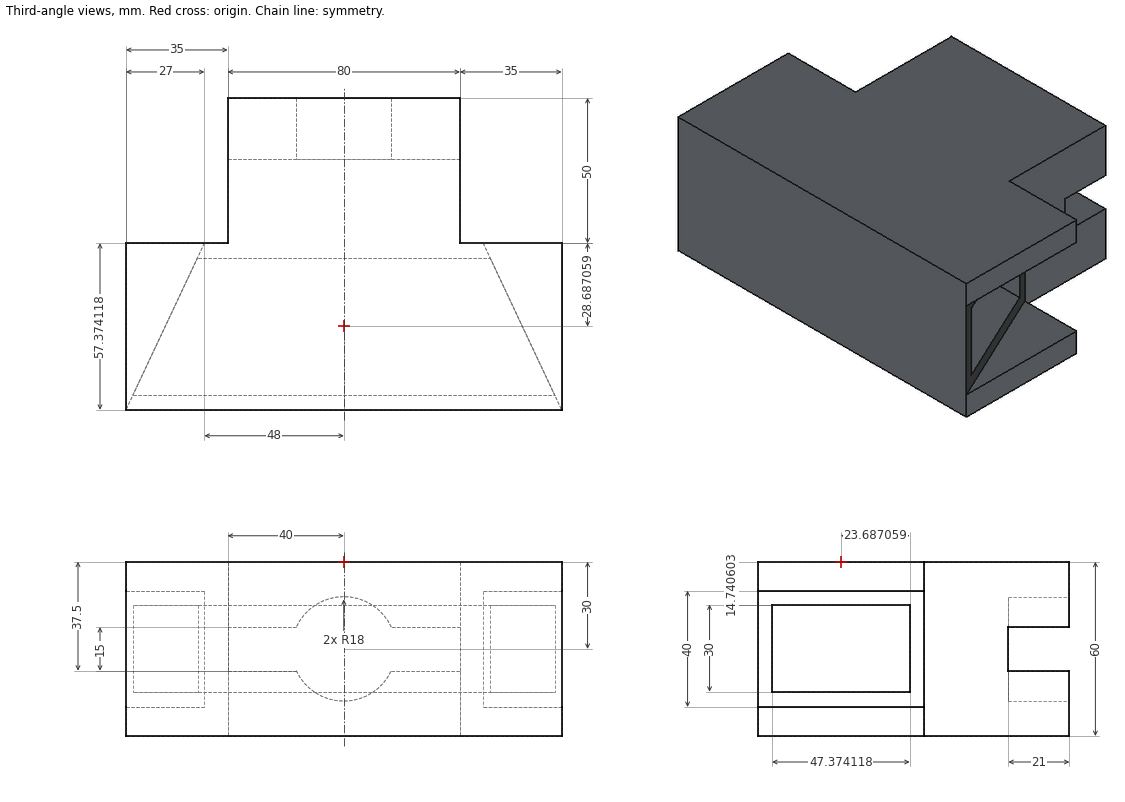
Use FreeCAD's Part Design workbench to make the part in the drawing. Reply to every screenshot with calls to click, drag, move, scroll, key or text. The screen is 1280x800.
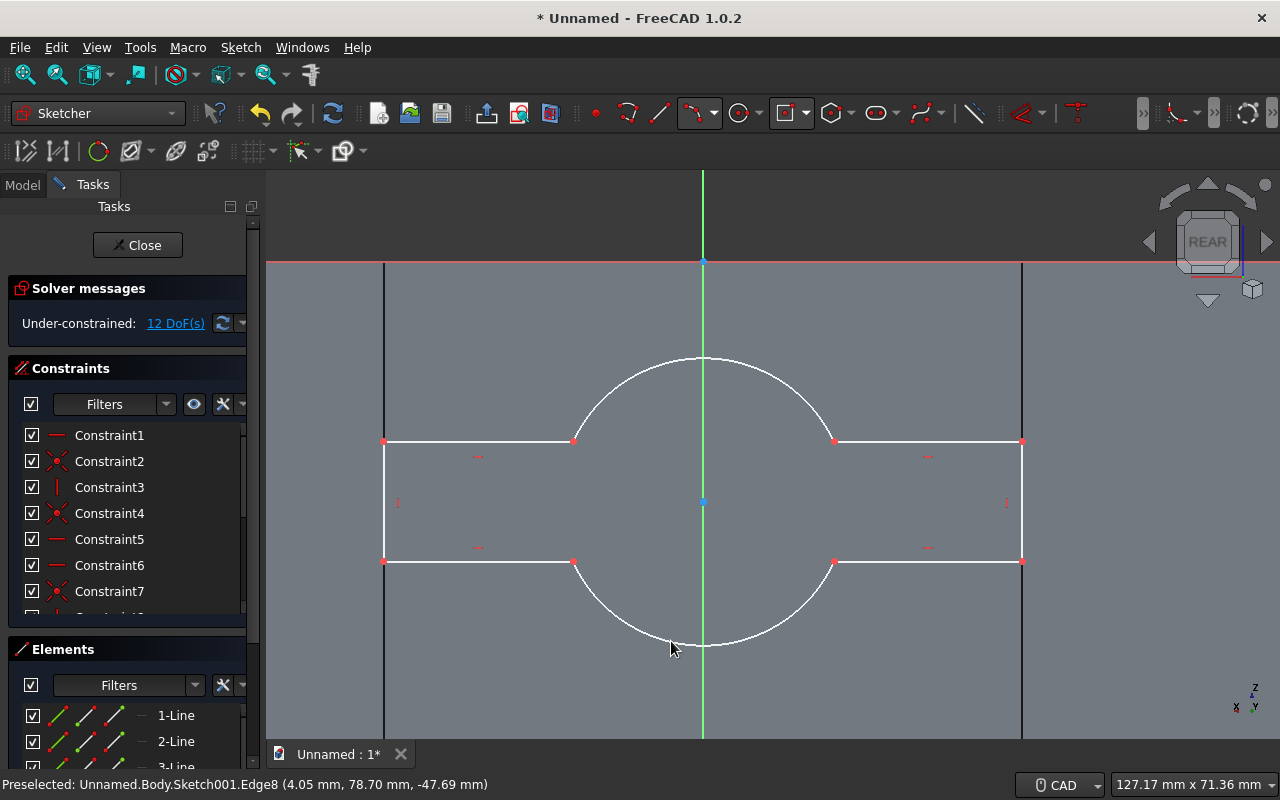
click(767, 373)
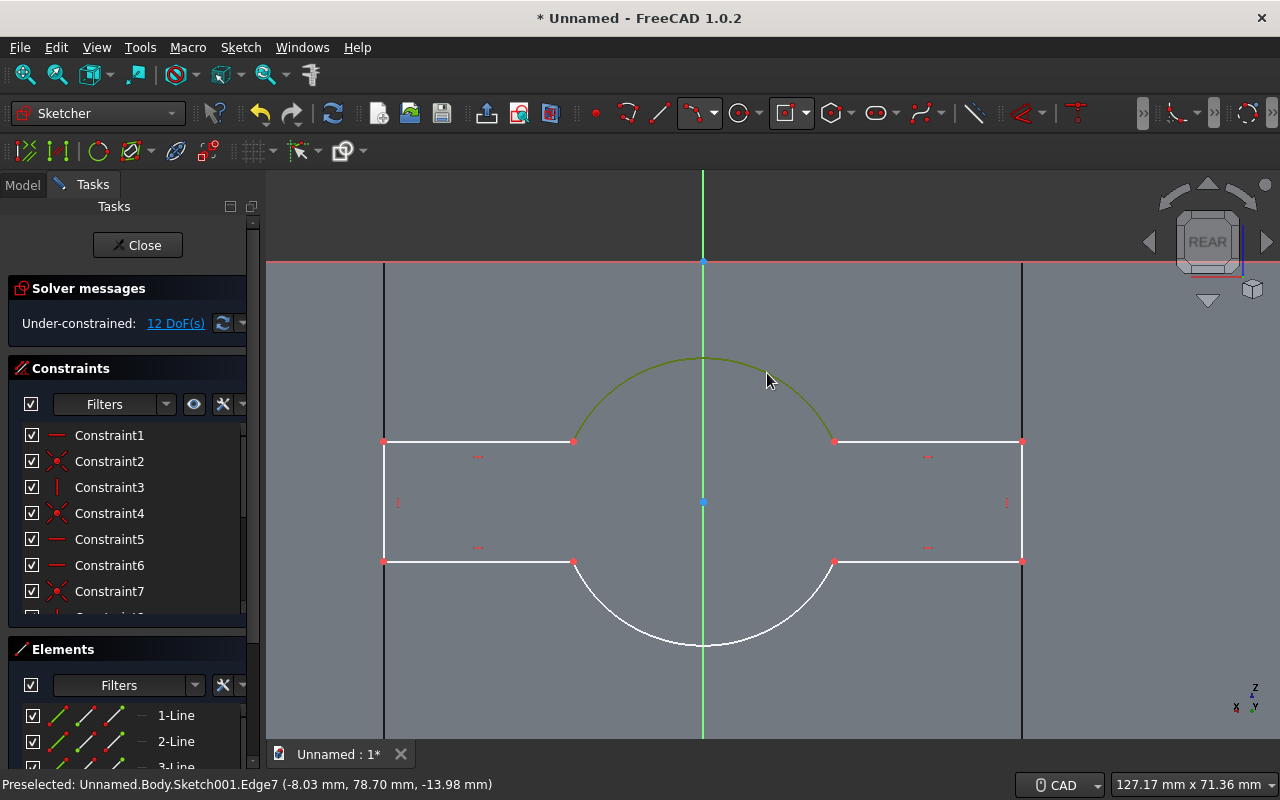
click(640, 631)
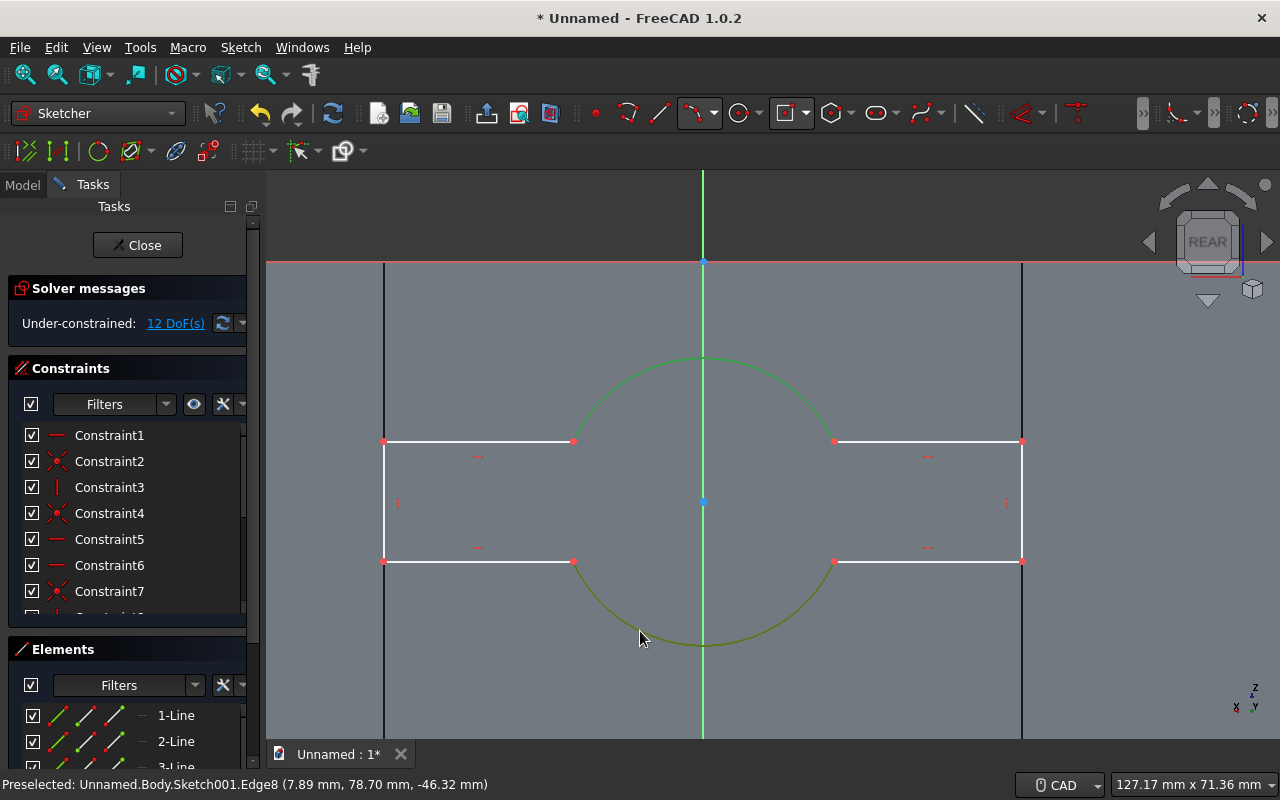
click(1076, 114)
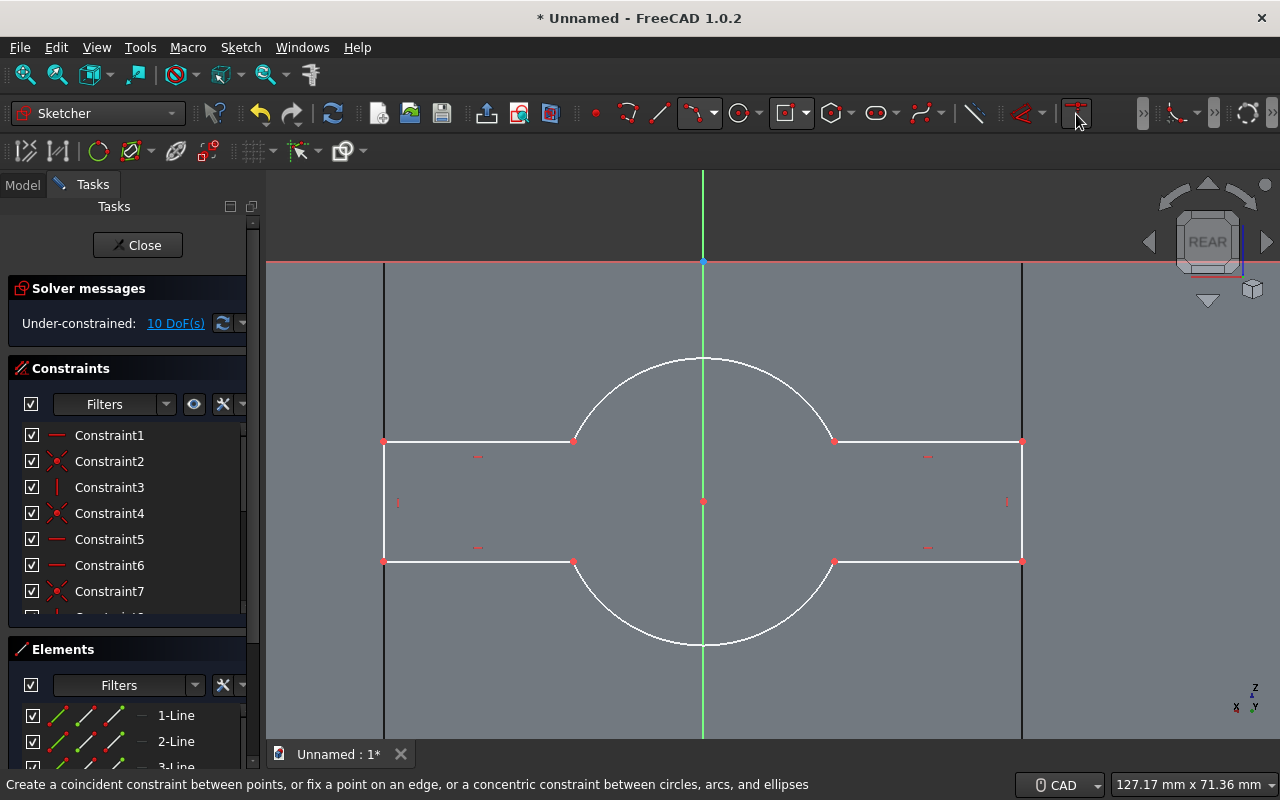
click(767, 373)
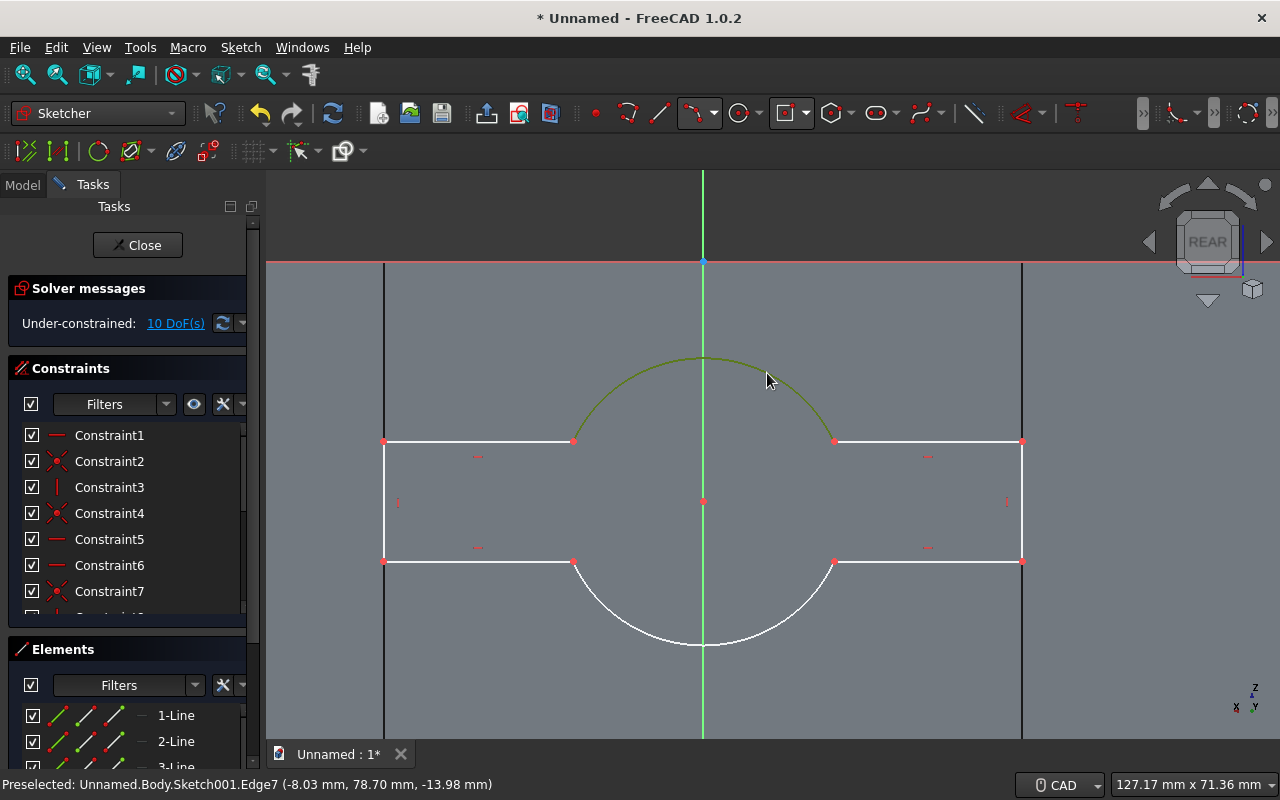
click(640, 631)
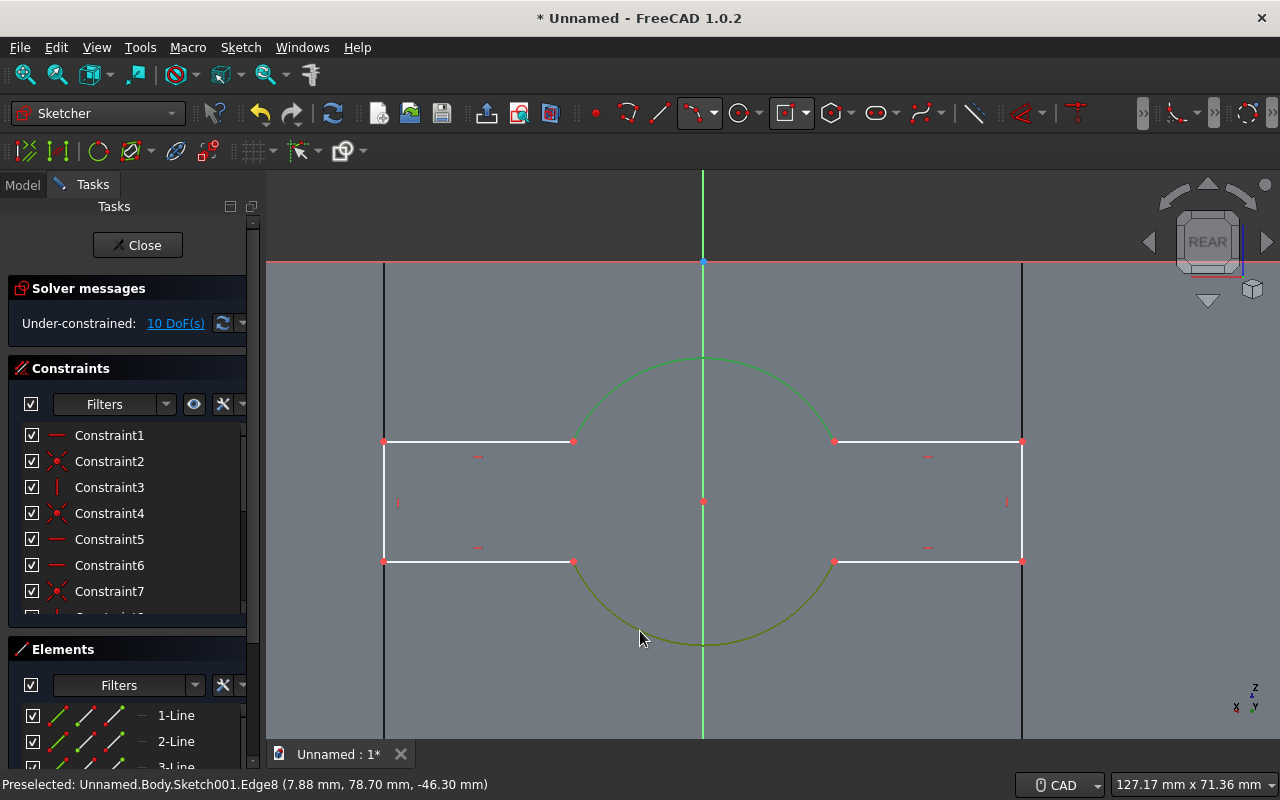
key(e)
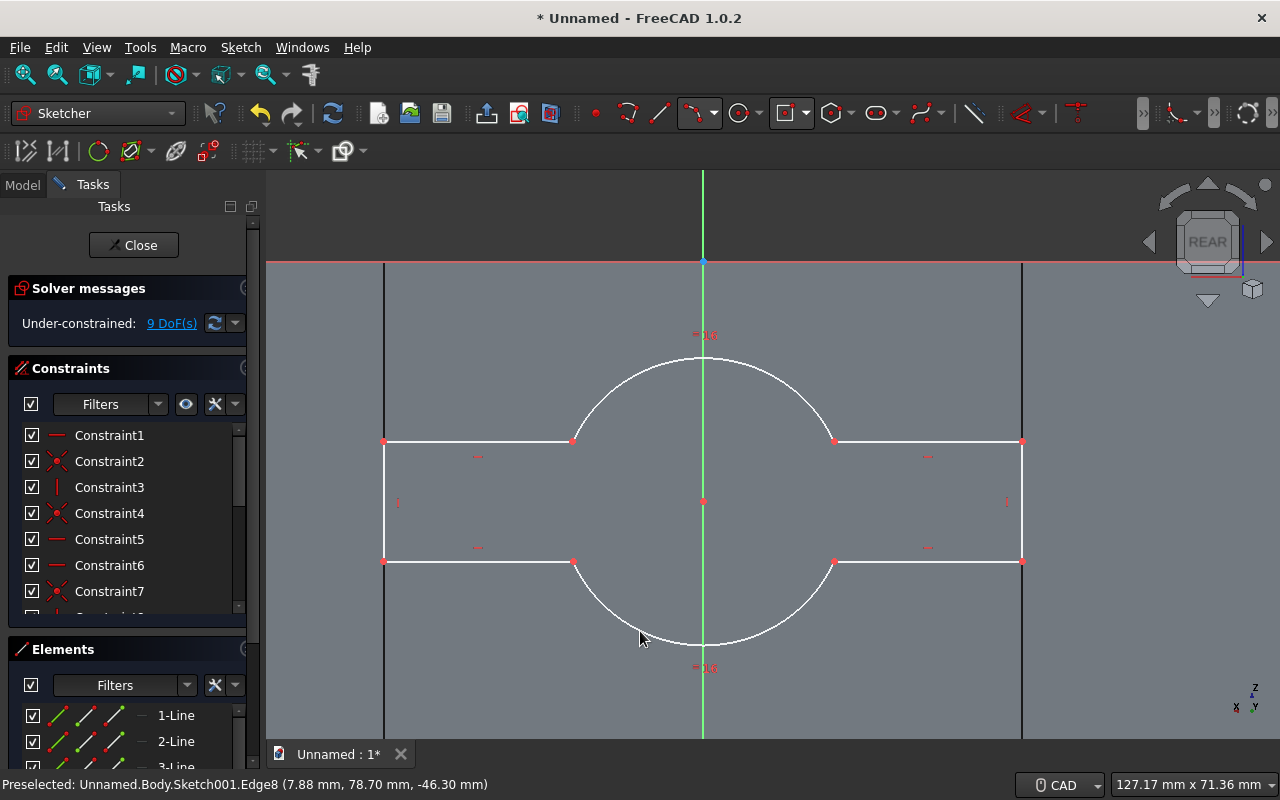
click(704, 502)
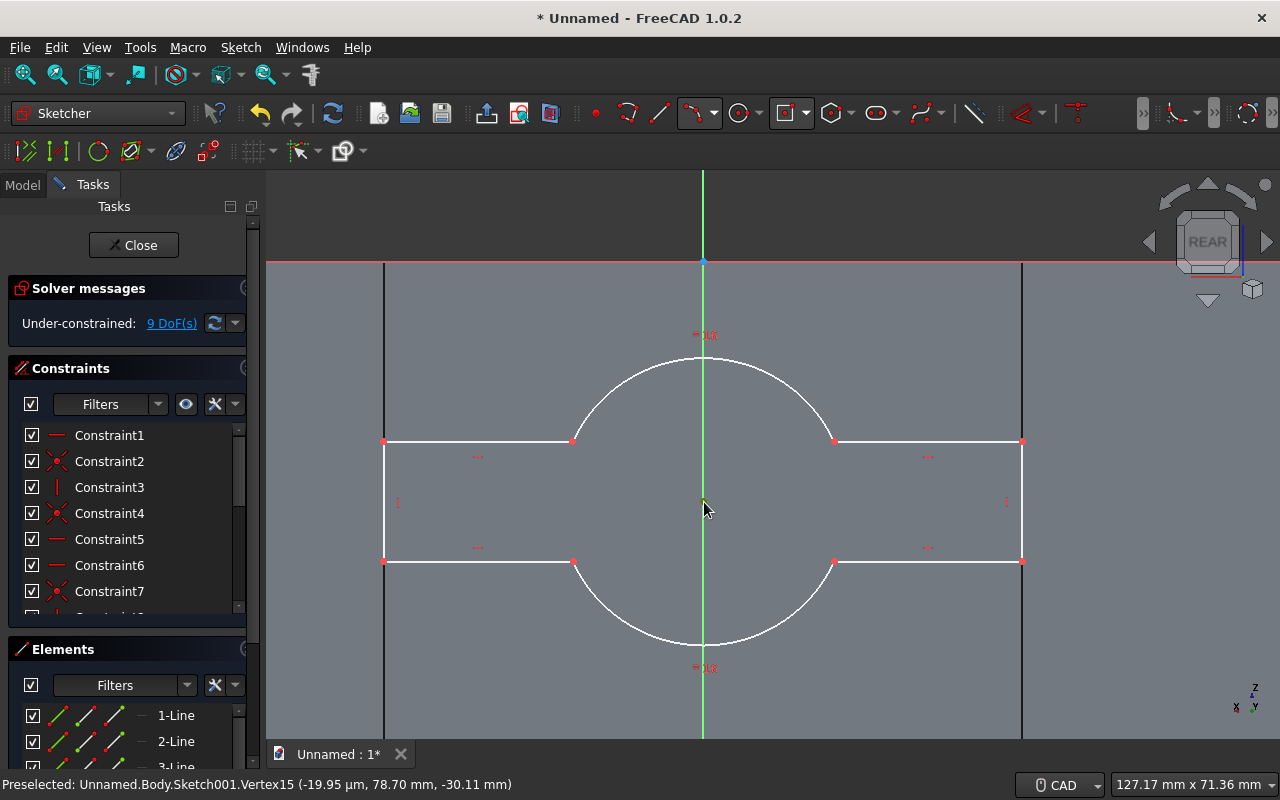
click(703, 601)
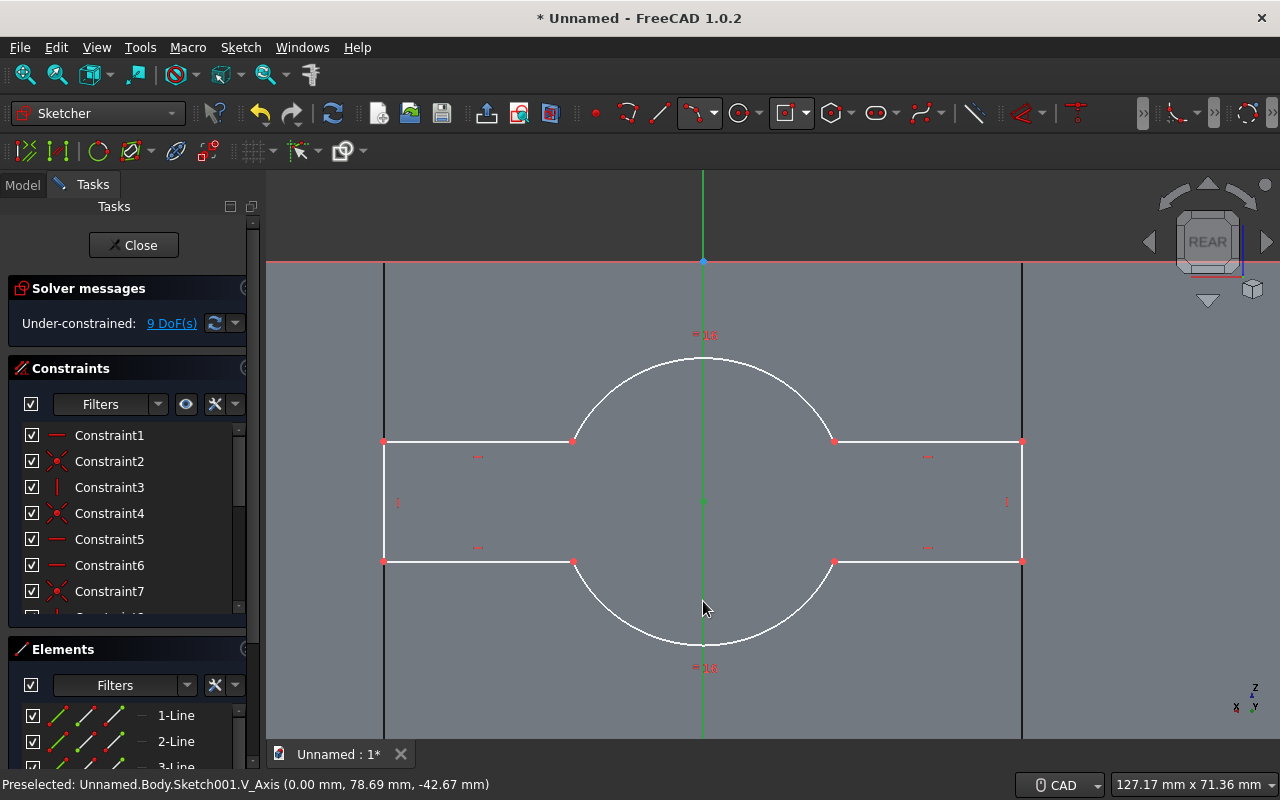
key(c)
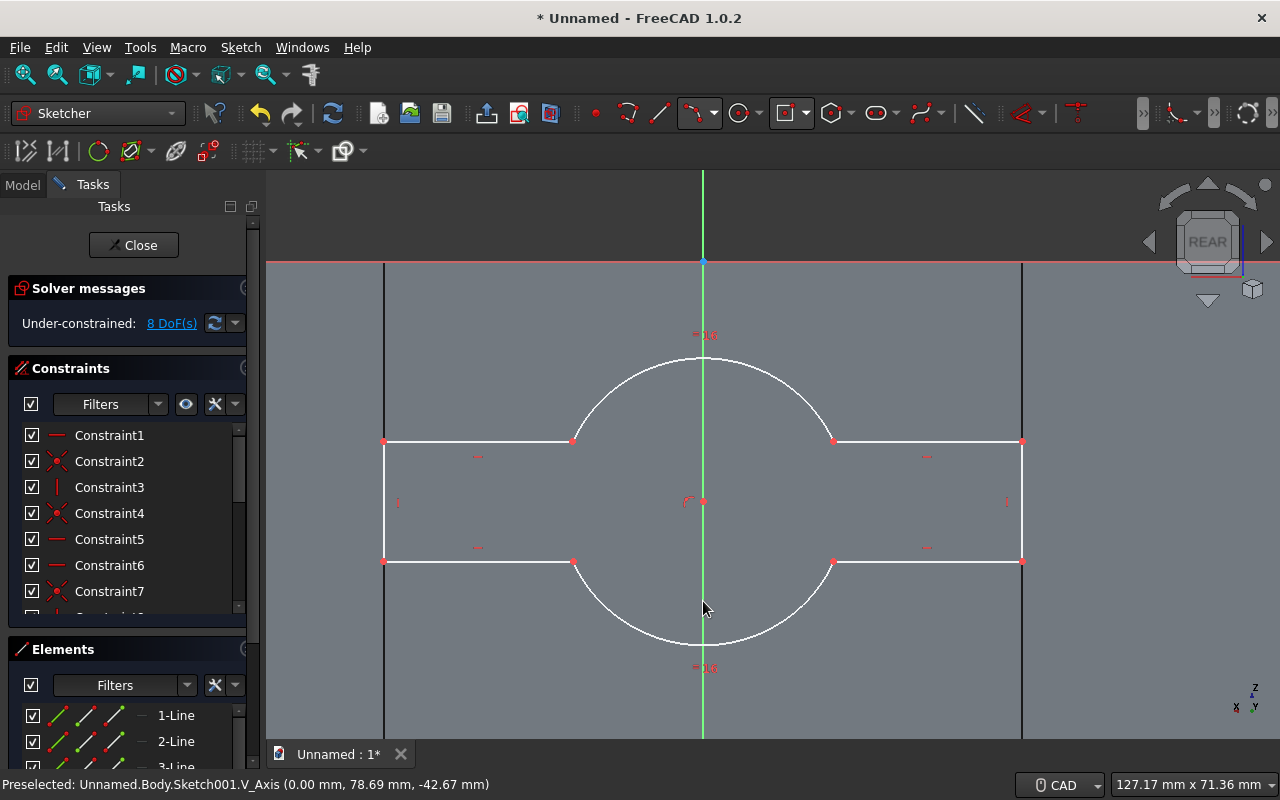
click(1022, 442)